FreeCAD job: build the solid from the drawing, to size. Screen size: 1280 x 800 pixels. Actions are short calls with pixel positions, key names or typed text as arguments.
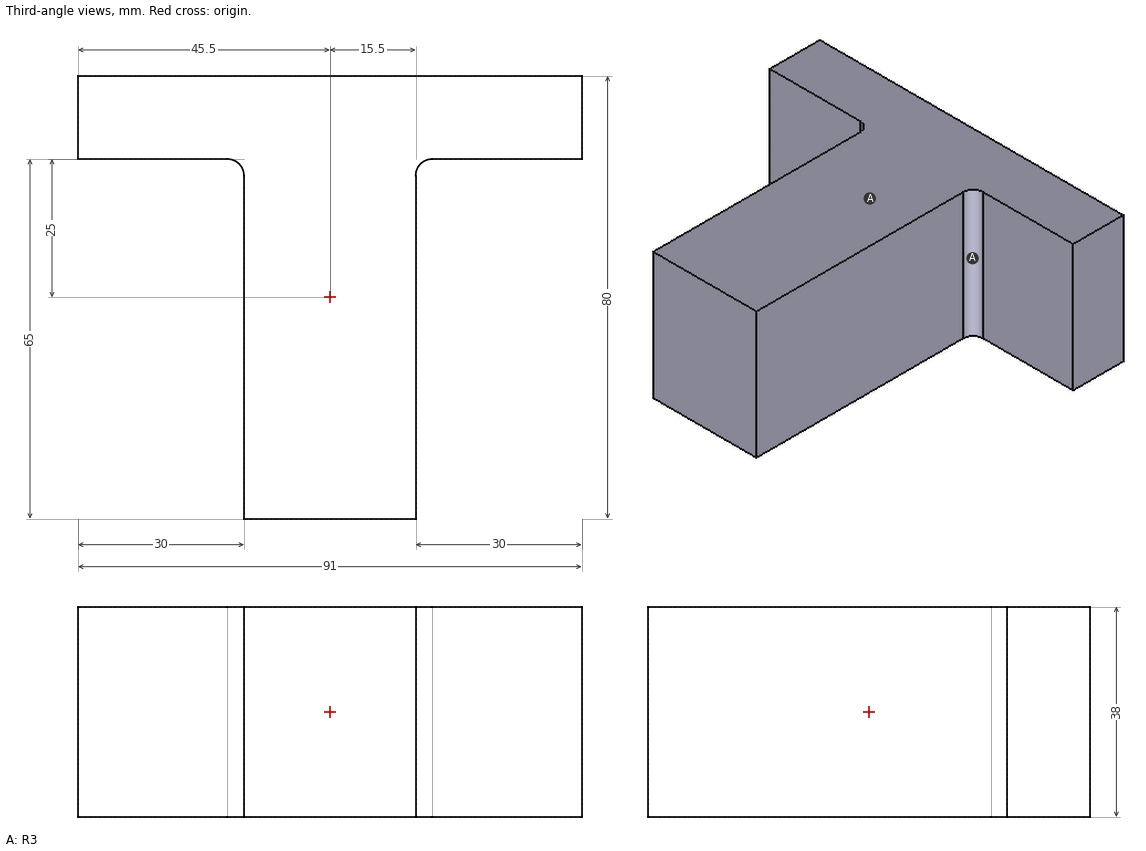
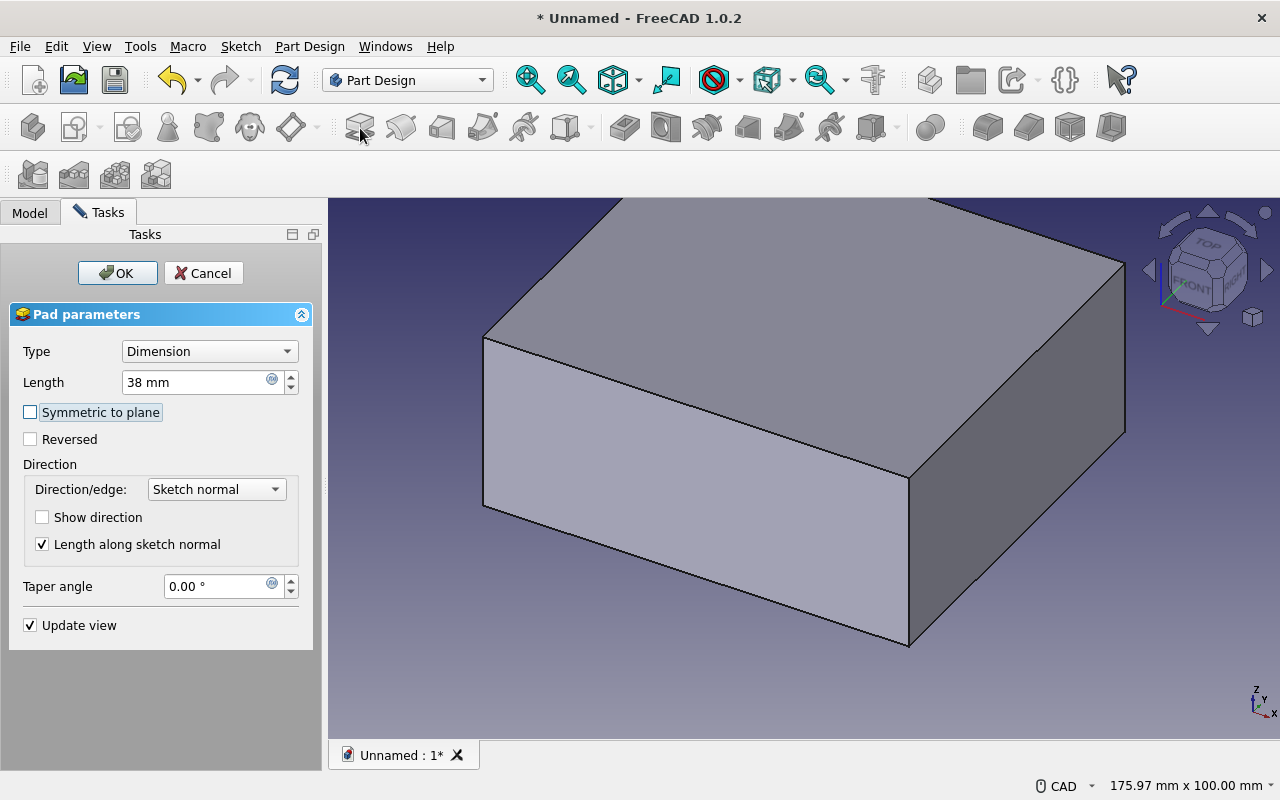
click(31, 412)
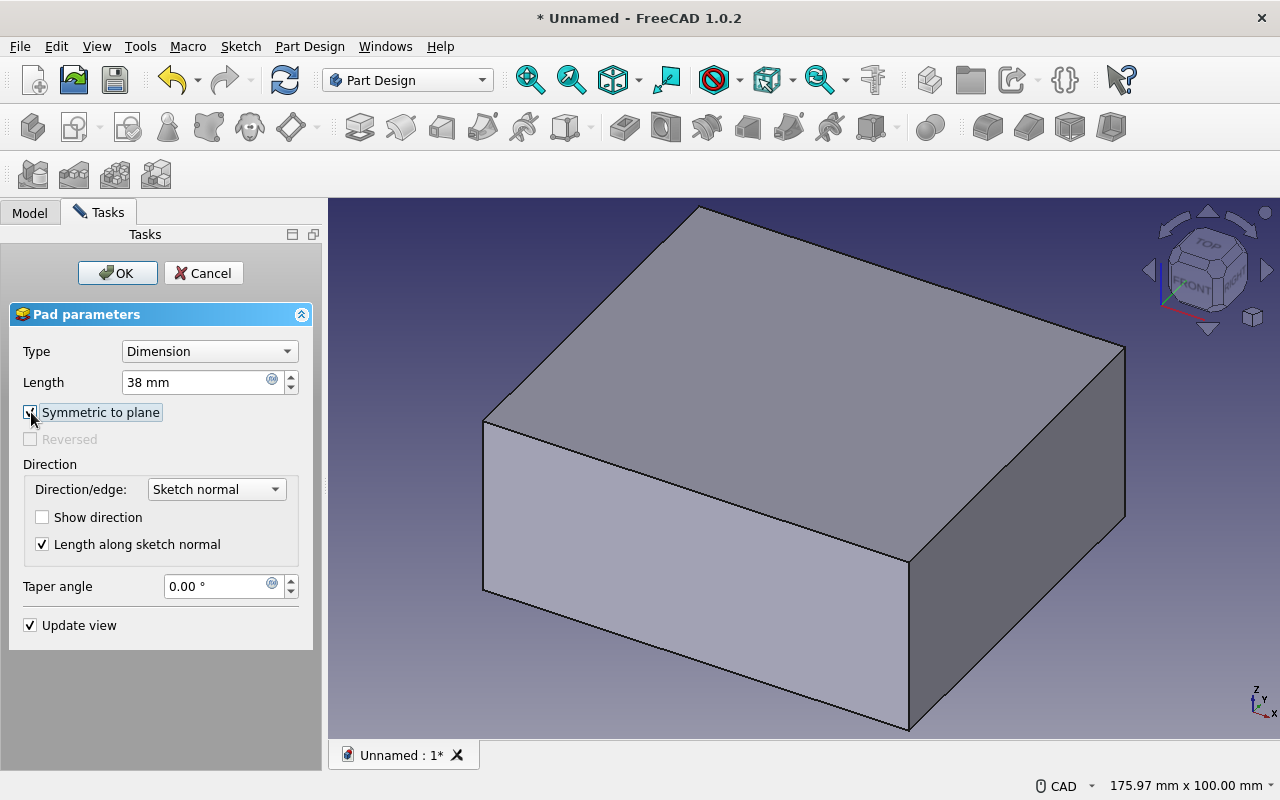
click(118, 273)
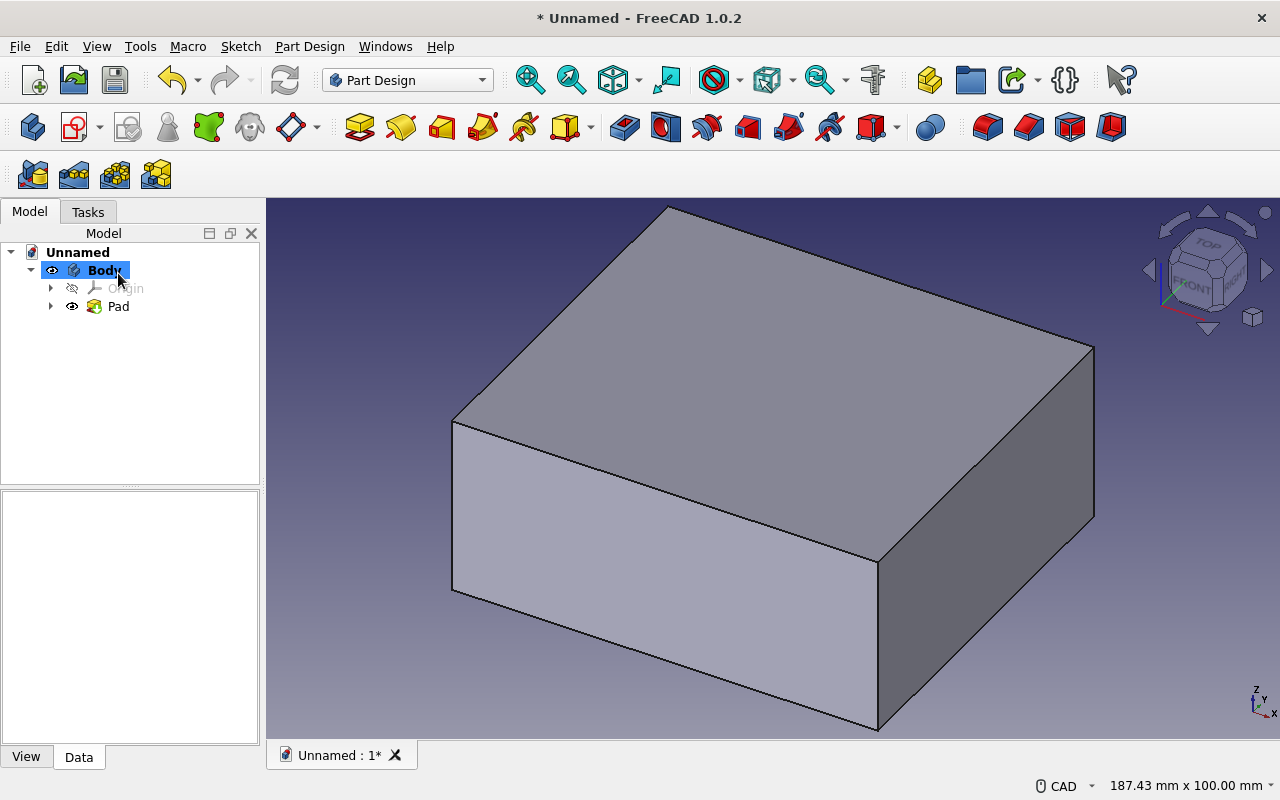
click(773, 383)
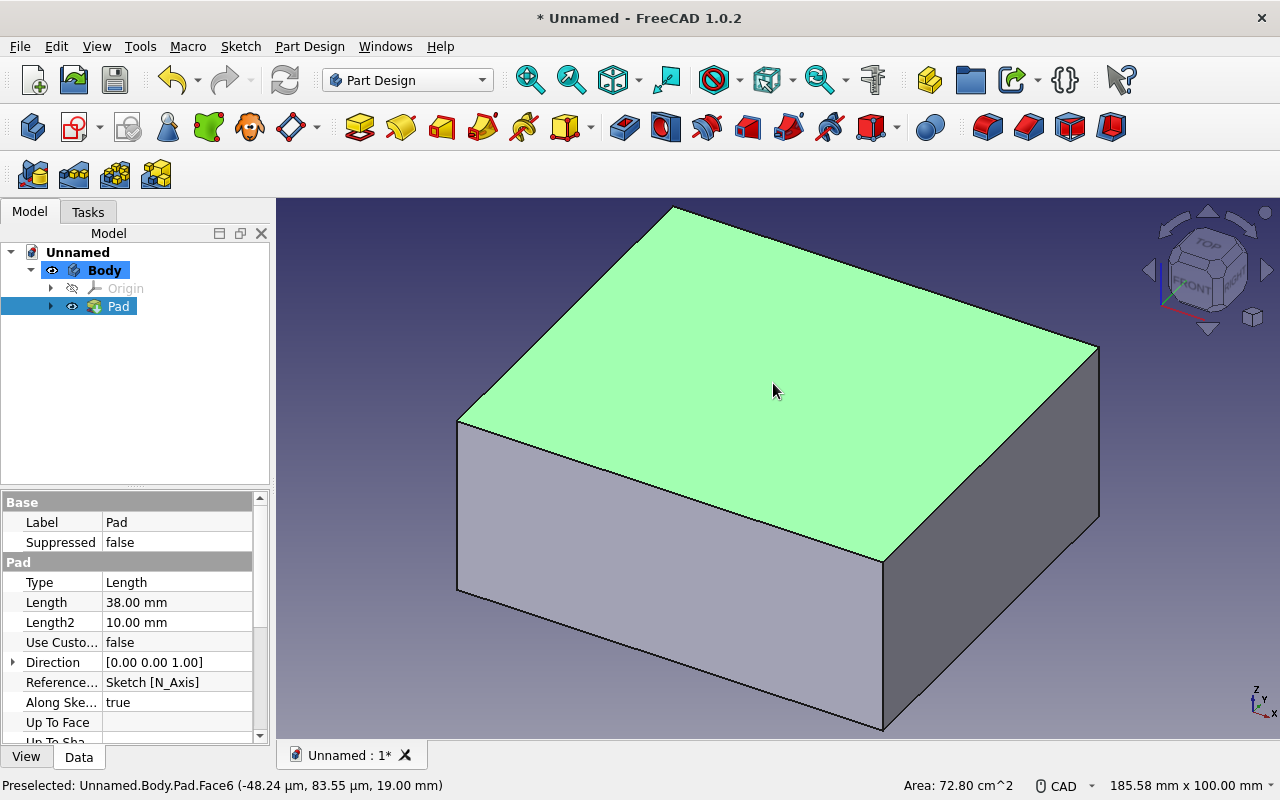
click(74, 128)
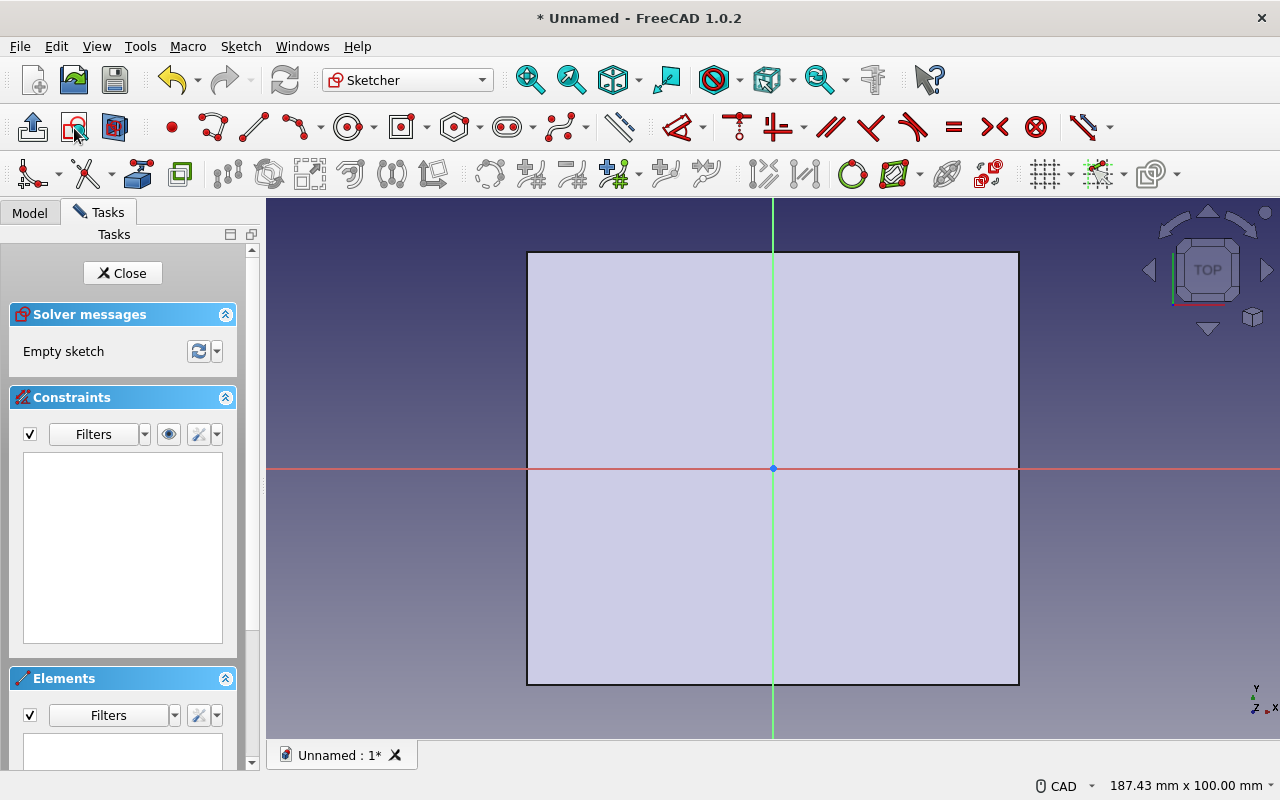
key(g)
key(r)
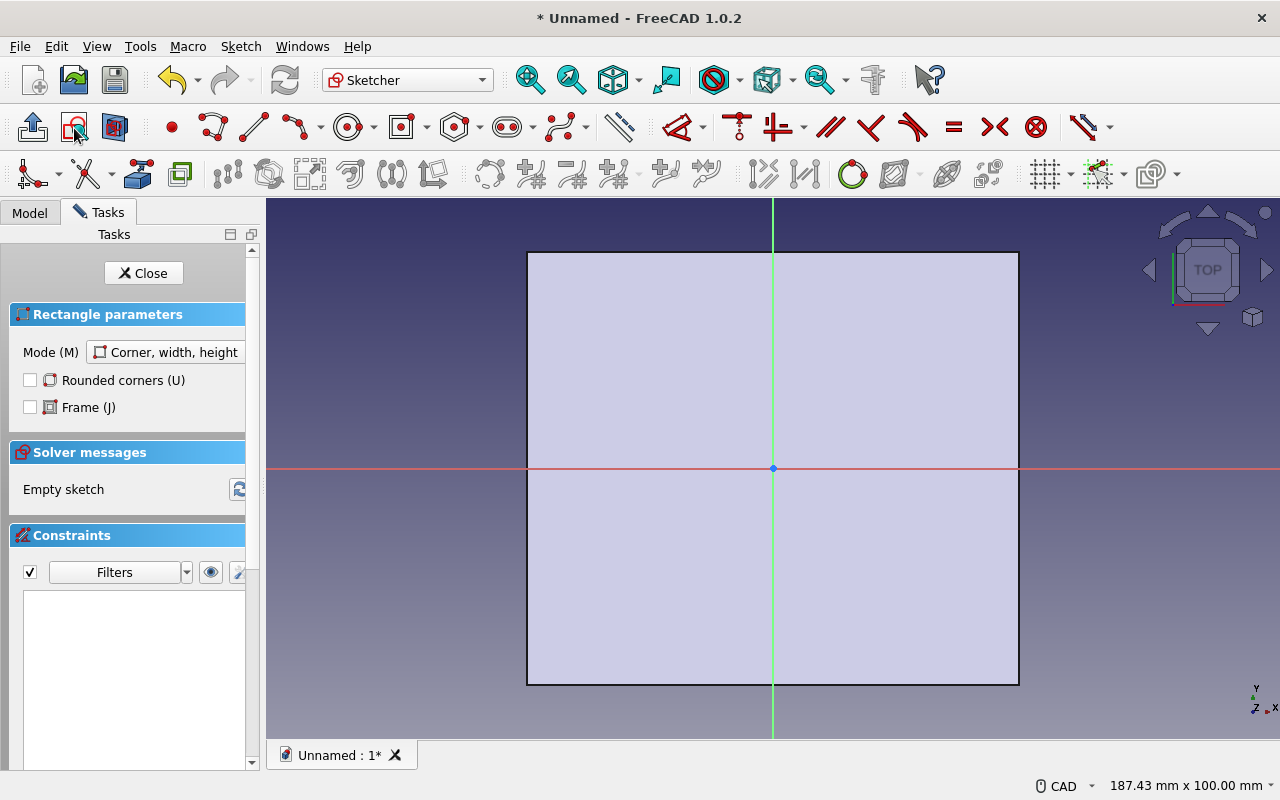
click(527, 333)
move(689, 685)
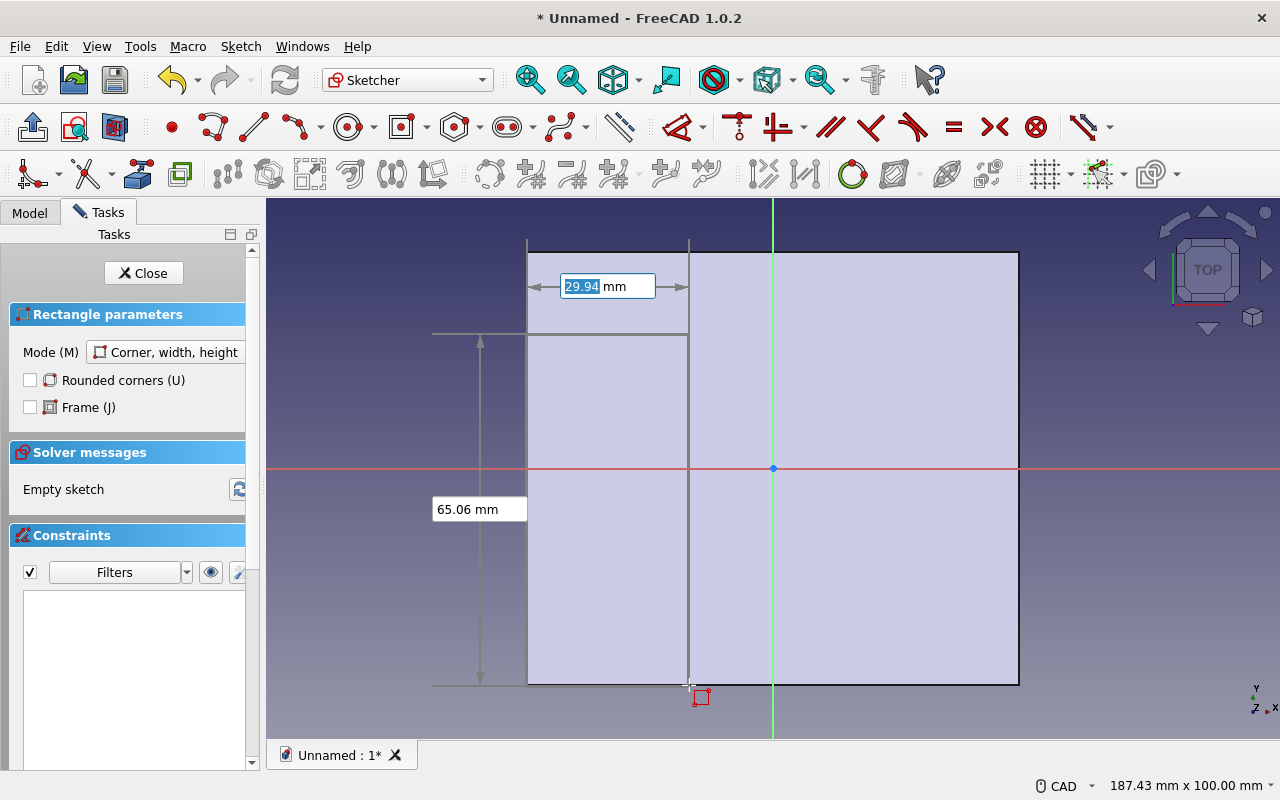
text(30)
key(Tab)
text(65)
key(Return)
key(Escape)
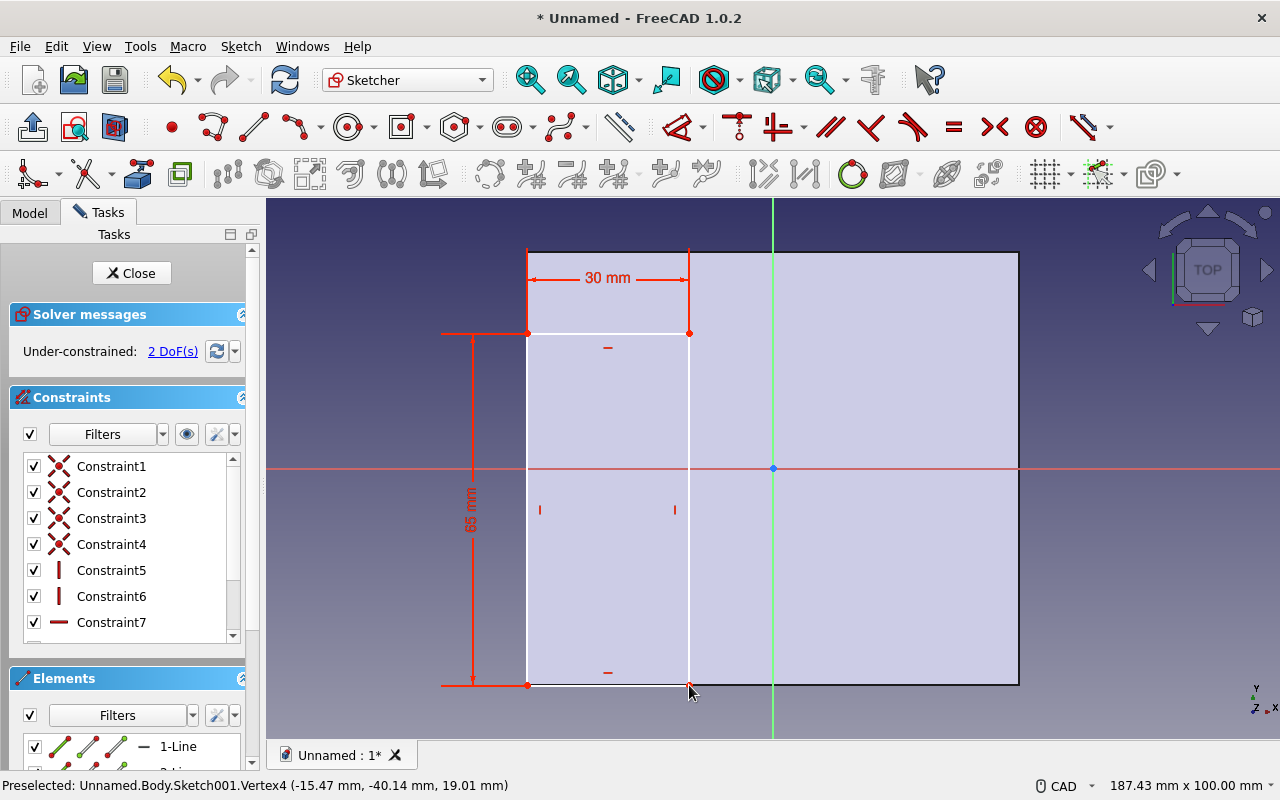
click(676, 128)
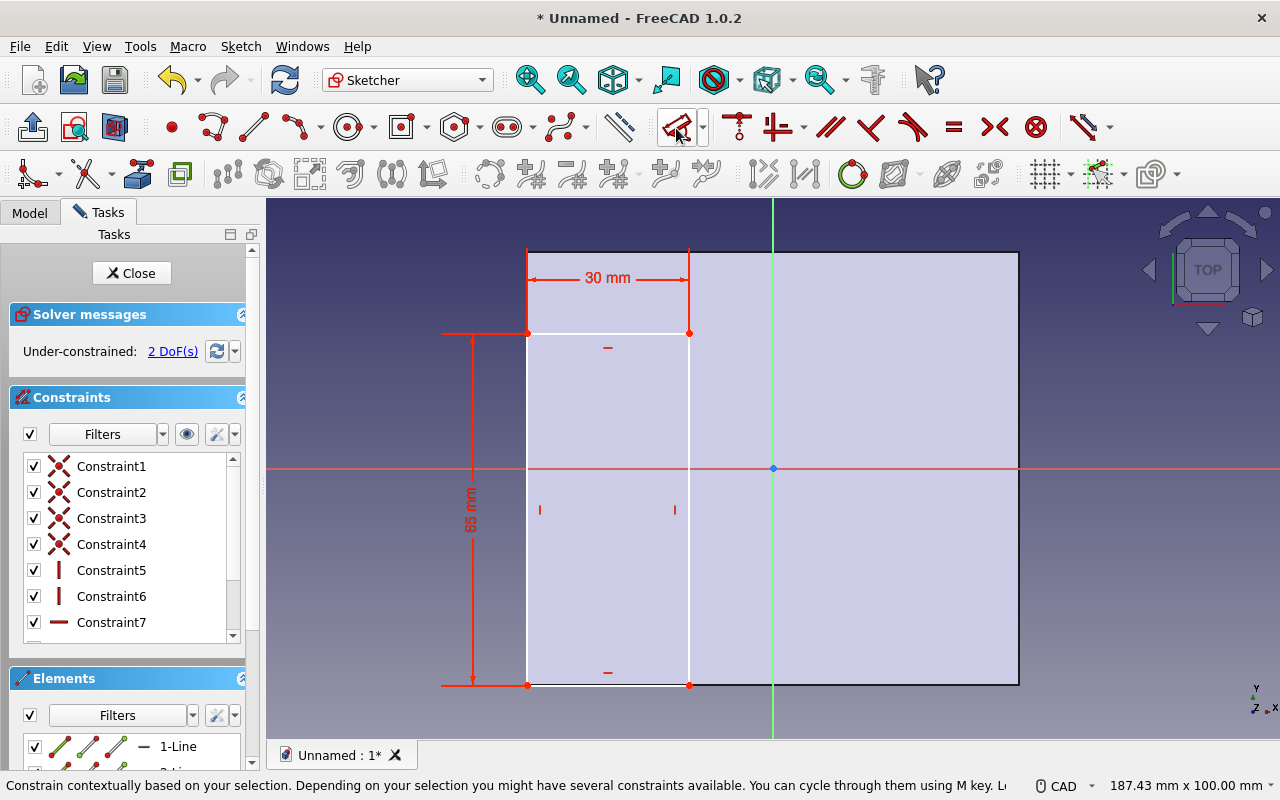
click(527, 334)
click(807, 401)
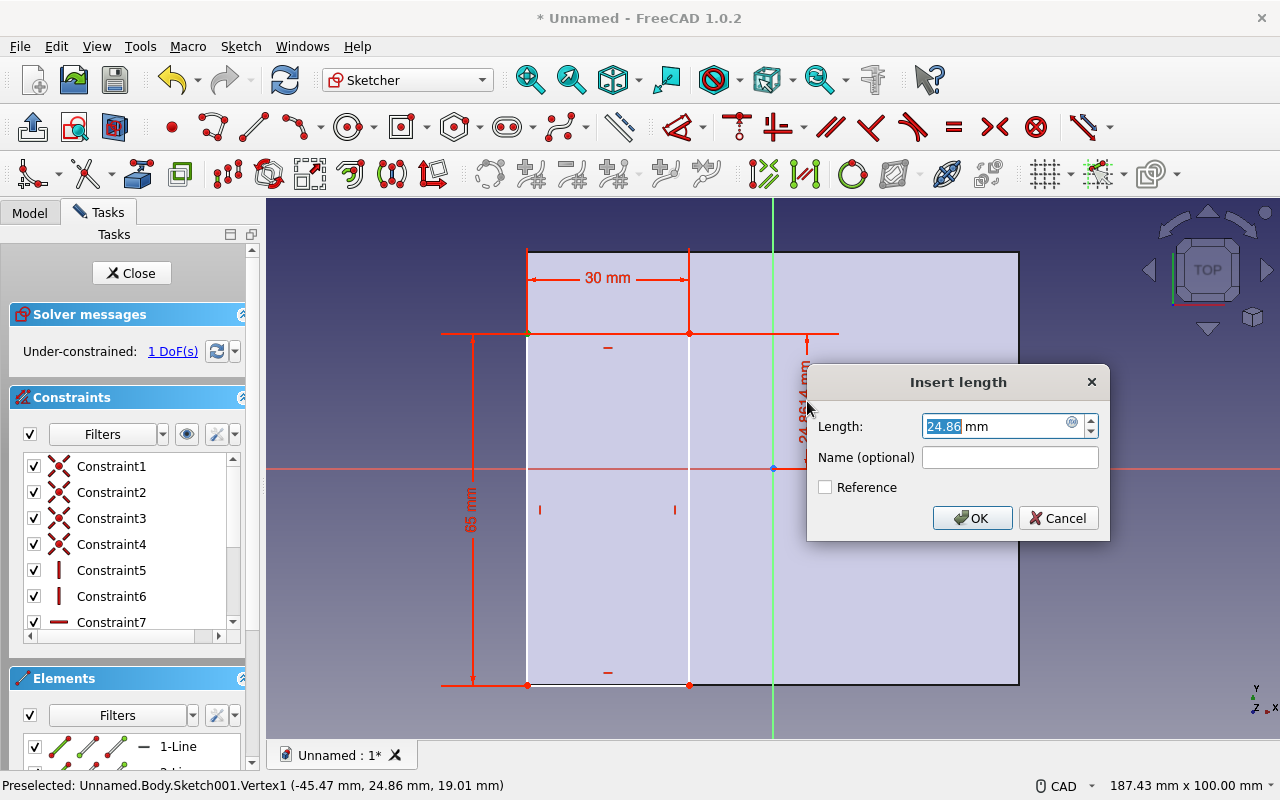
text(25)
key(Return)